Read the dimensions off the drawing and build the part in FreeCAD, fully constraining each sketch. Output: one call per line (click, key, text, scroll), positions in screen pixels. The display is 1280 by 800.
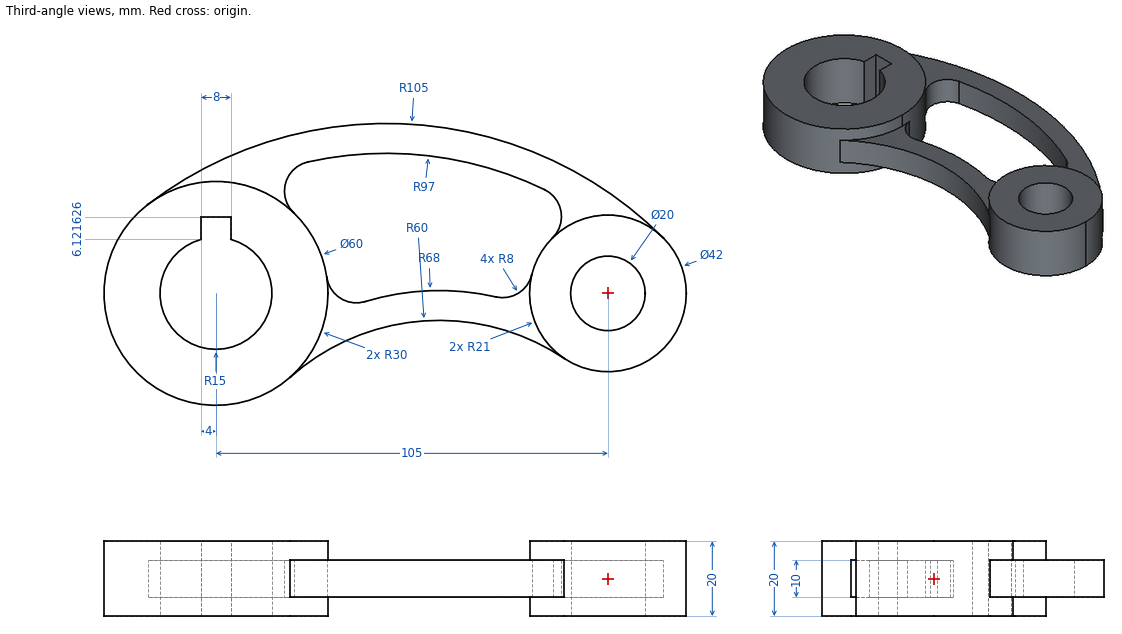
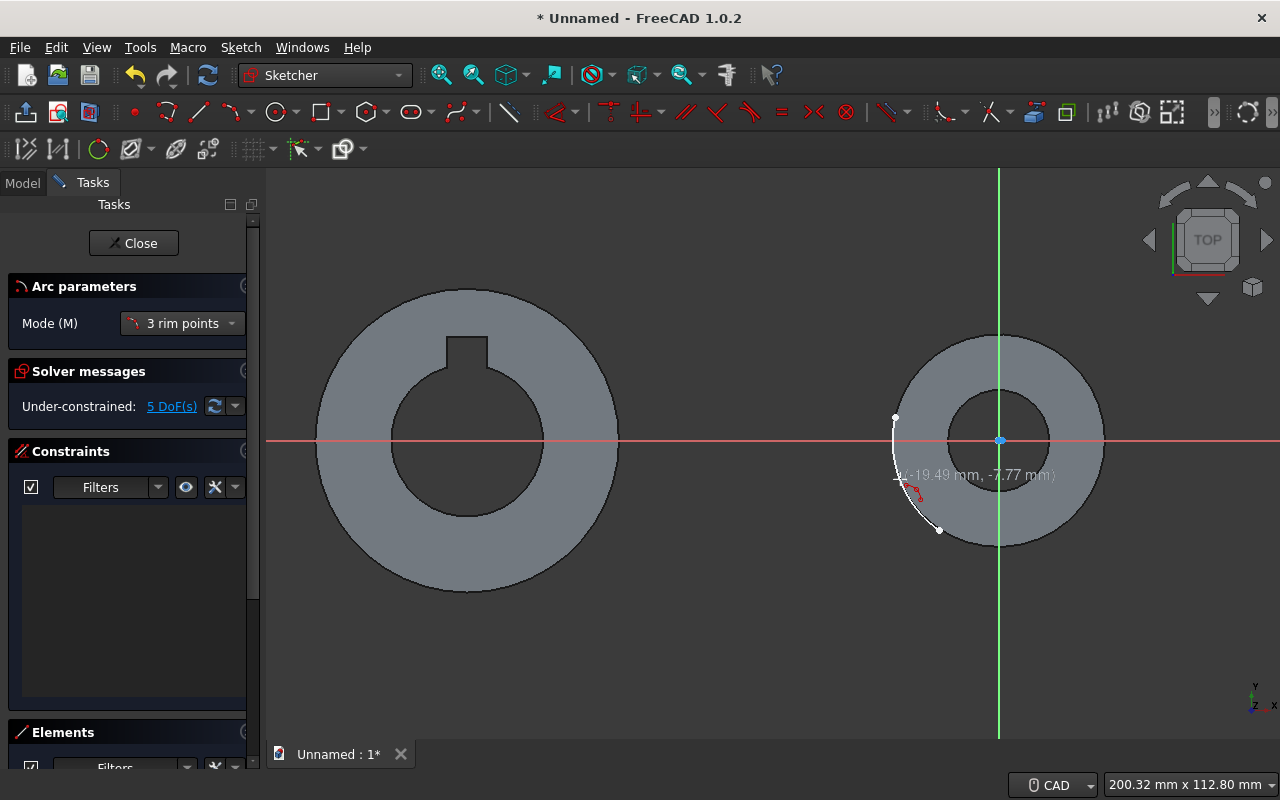
click(895, 418)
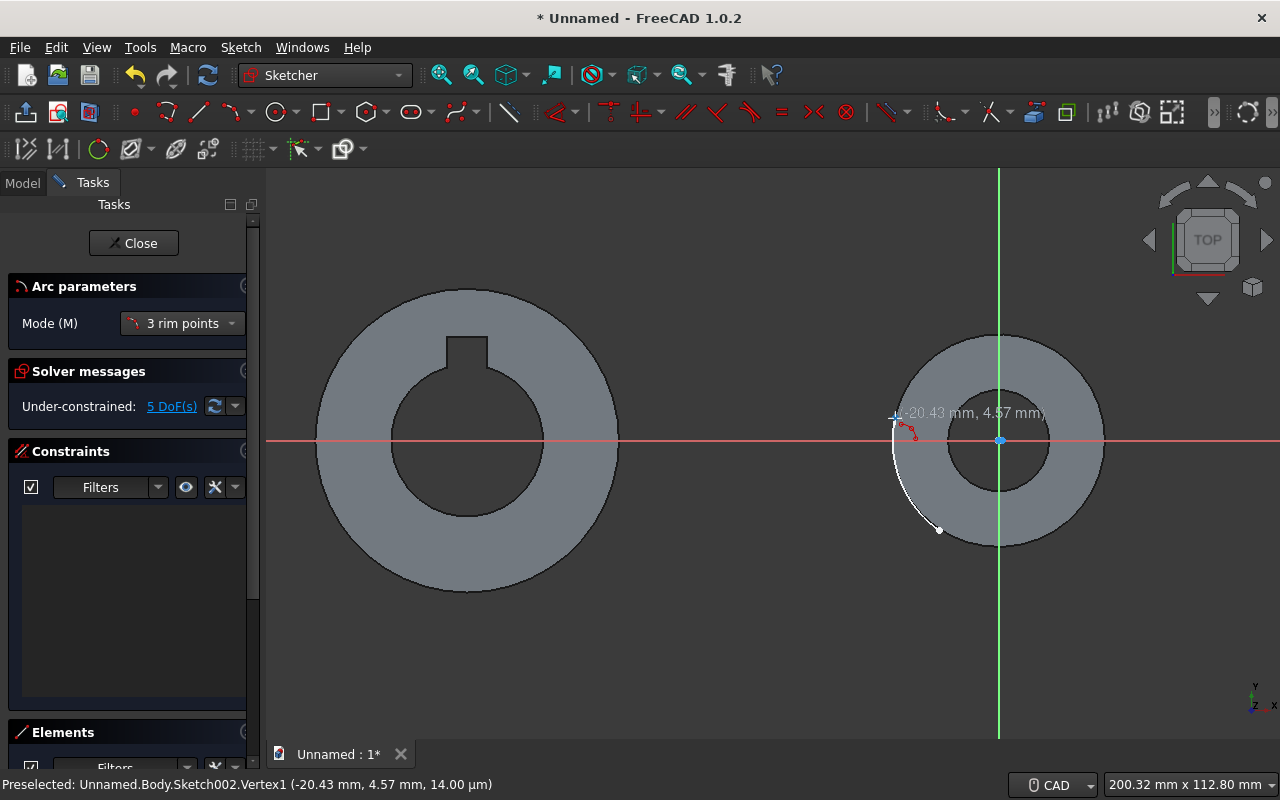
scroll(847, 446, up, 6)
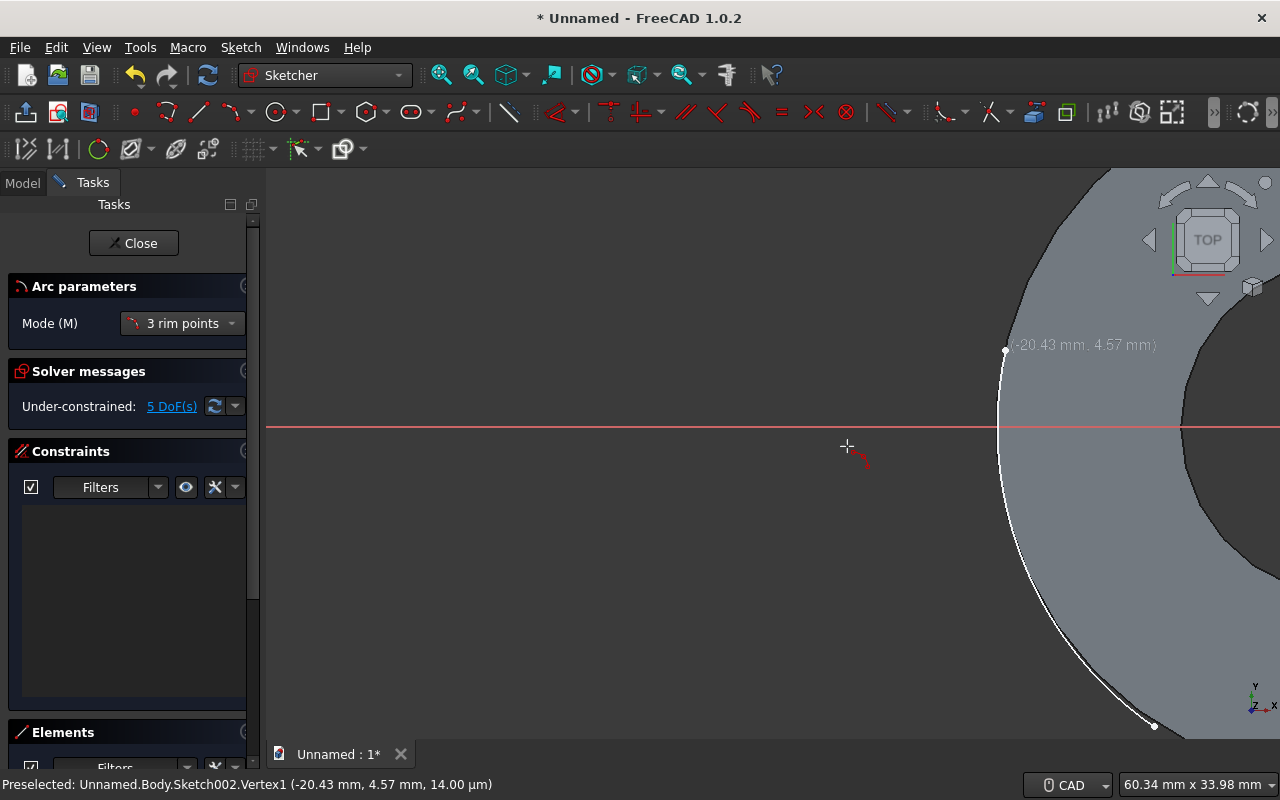
click(845, 443)
click(978, 399)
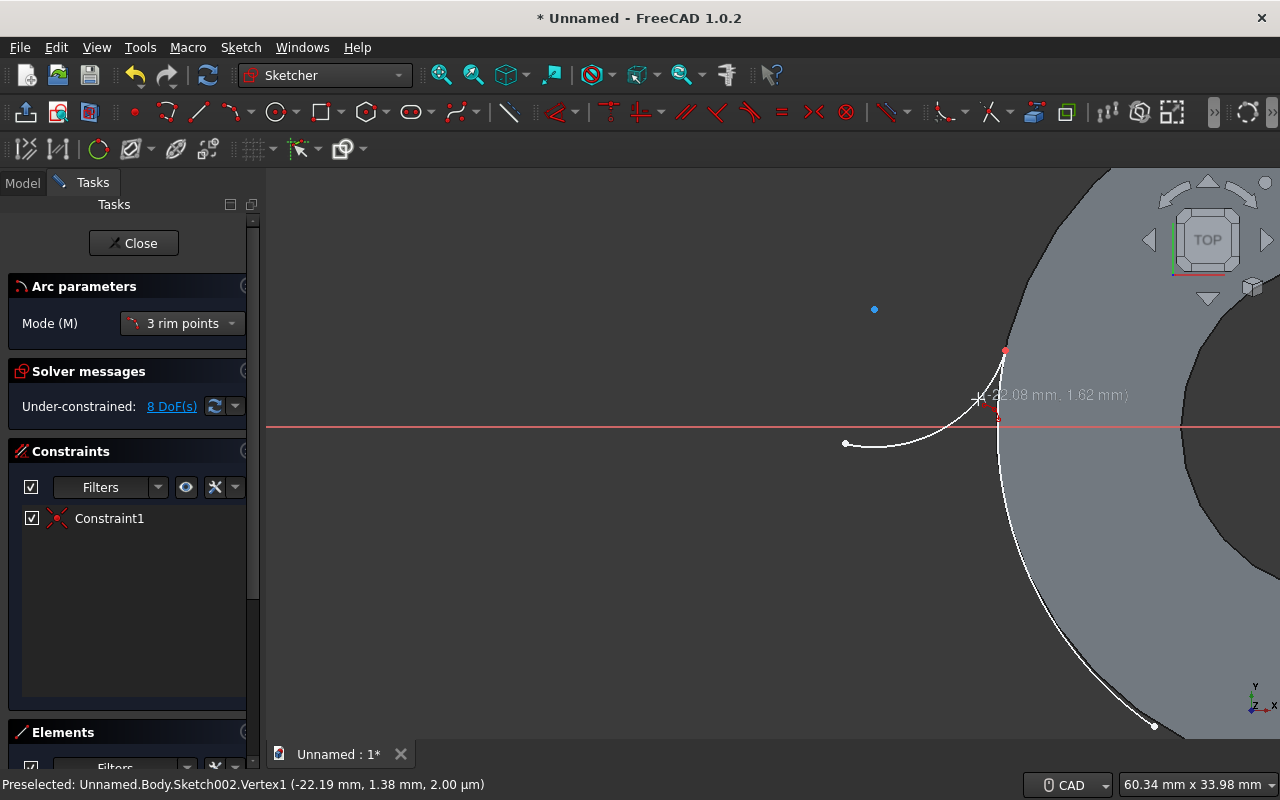
click(845, 444)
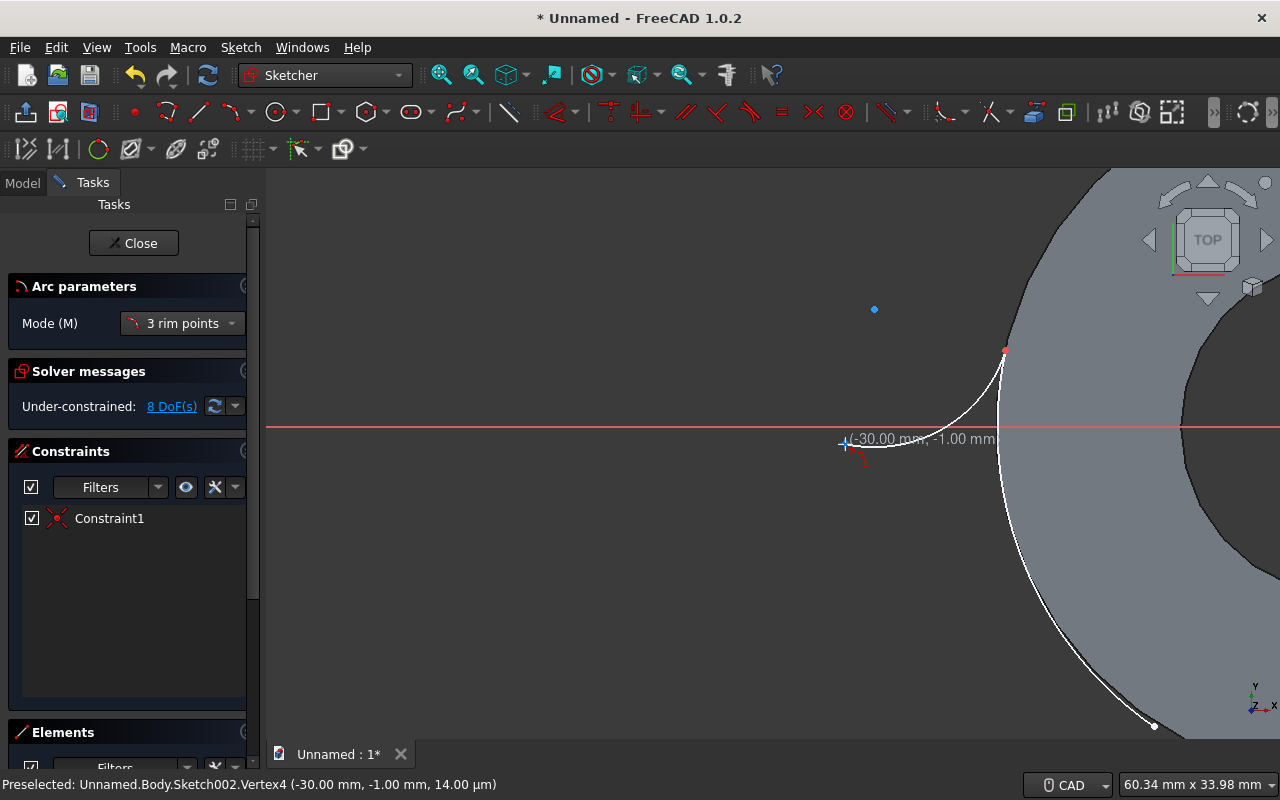
scroll(792, 525, down, 7)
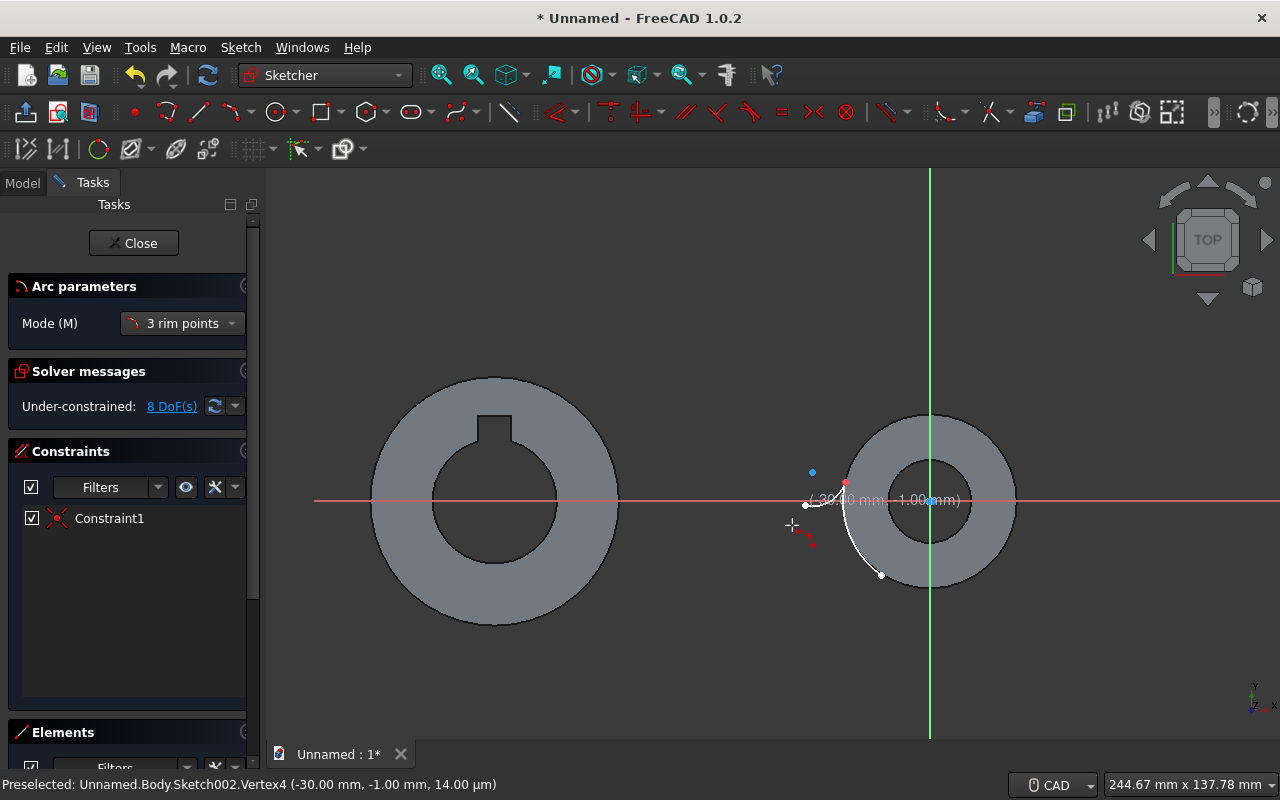
scroll(660, 511, up, 3)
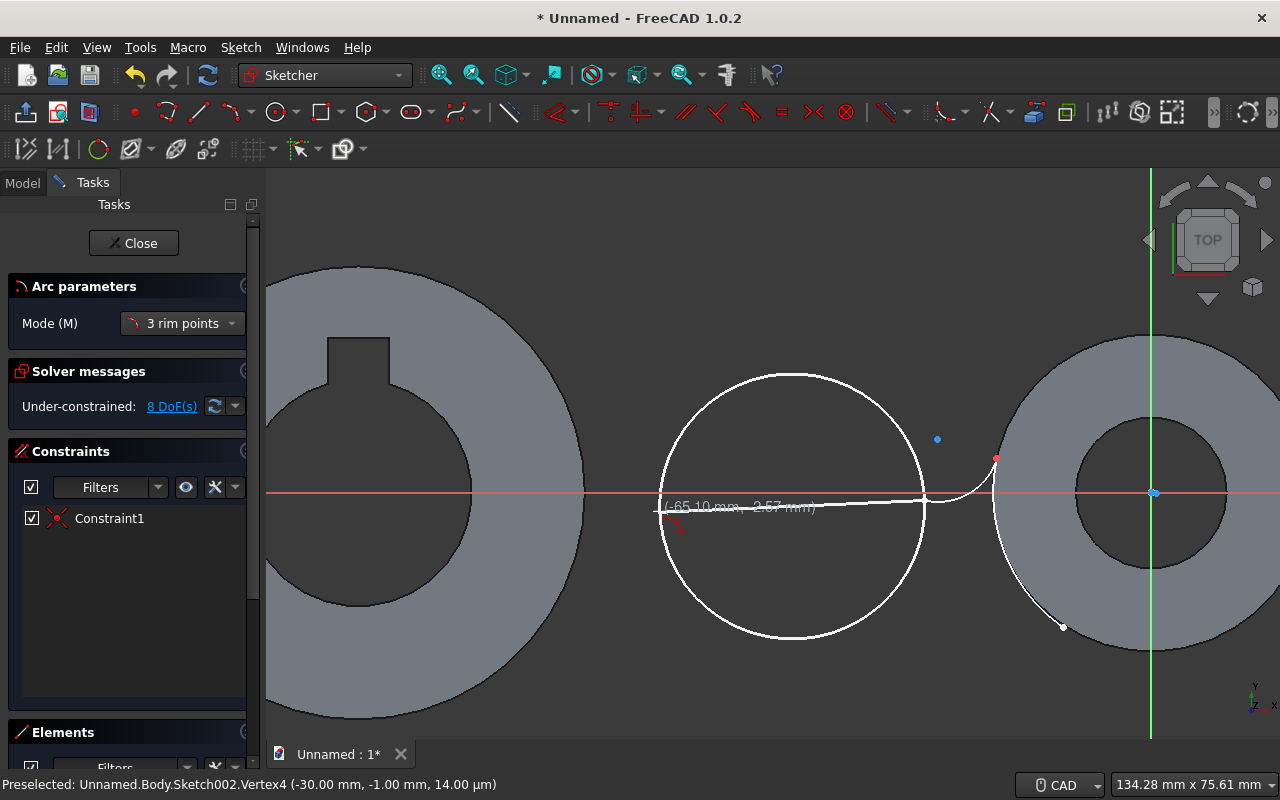
click(660, 510)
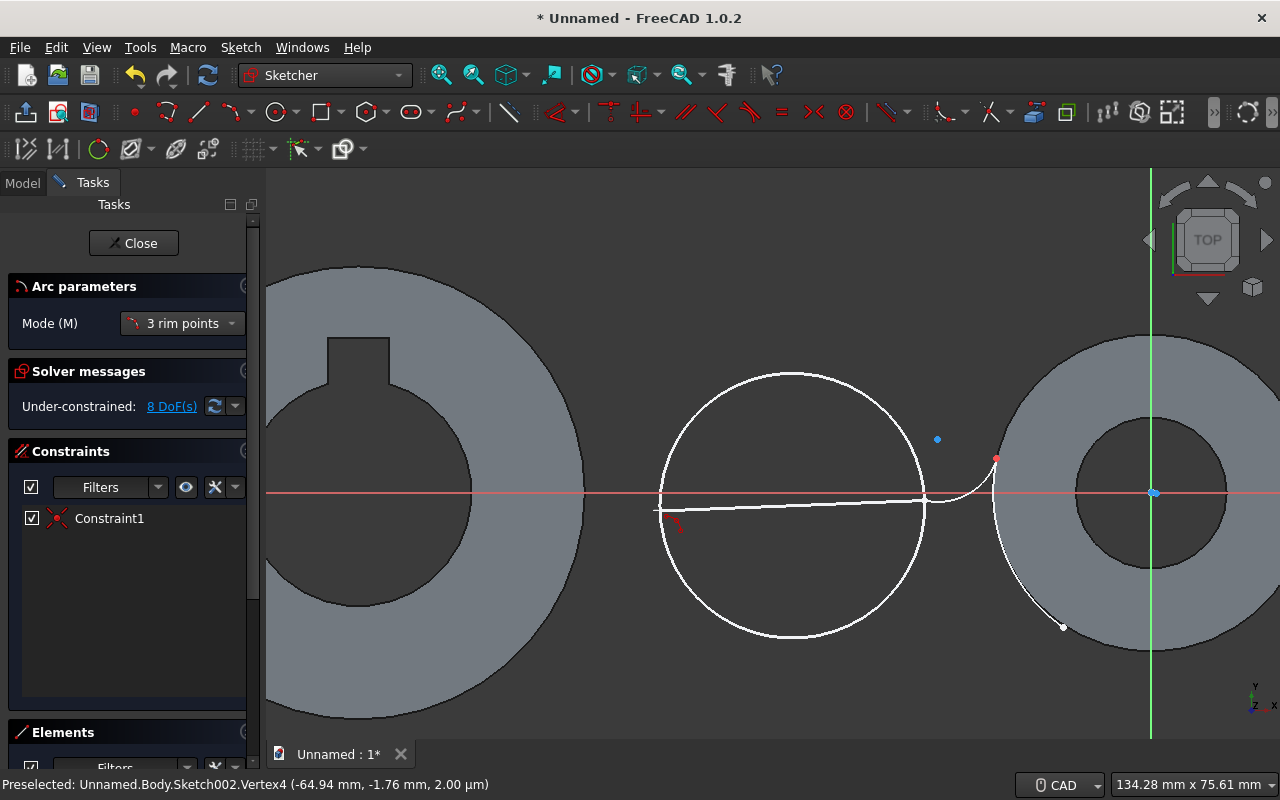
scroll(819, 487, up, 6)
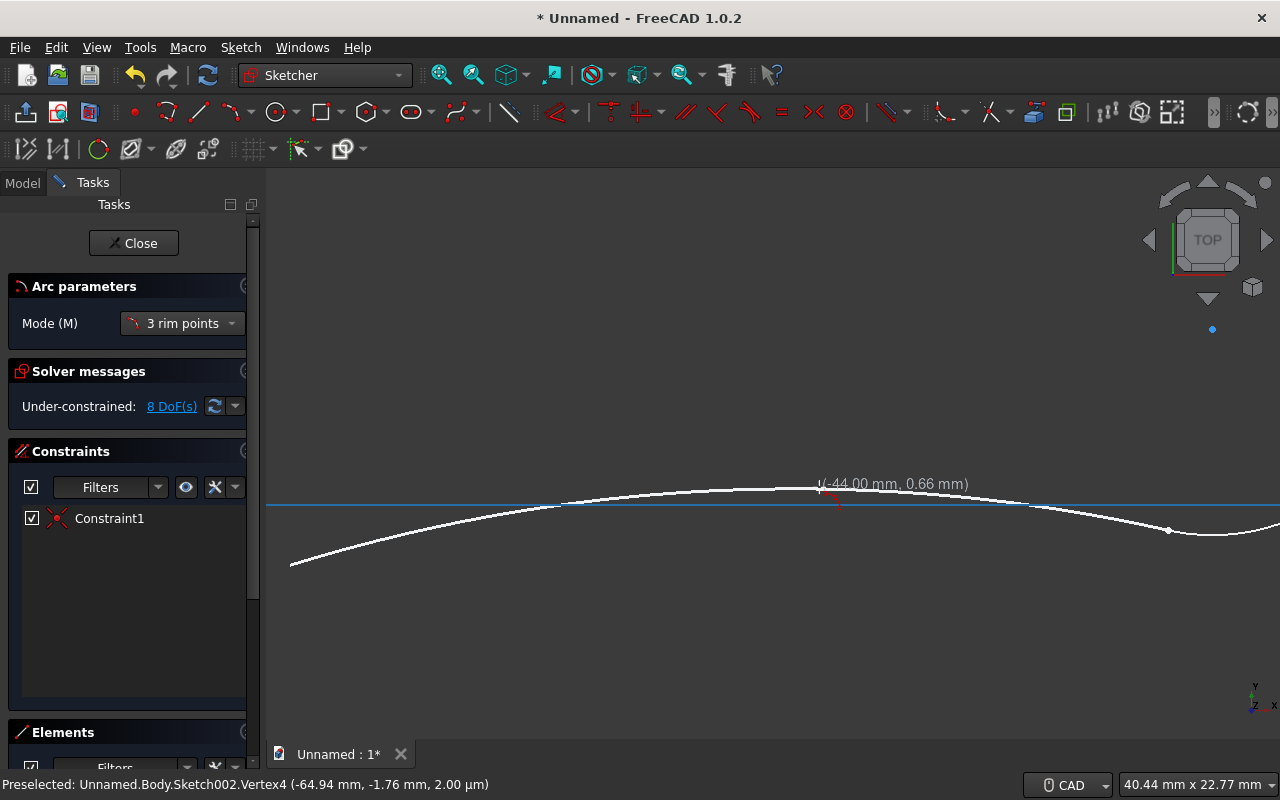
click(817, 487)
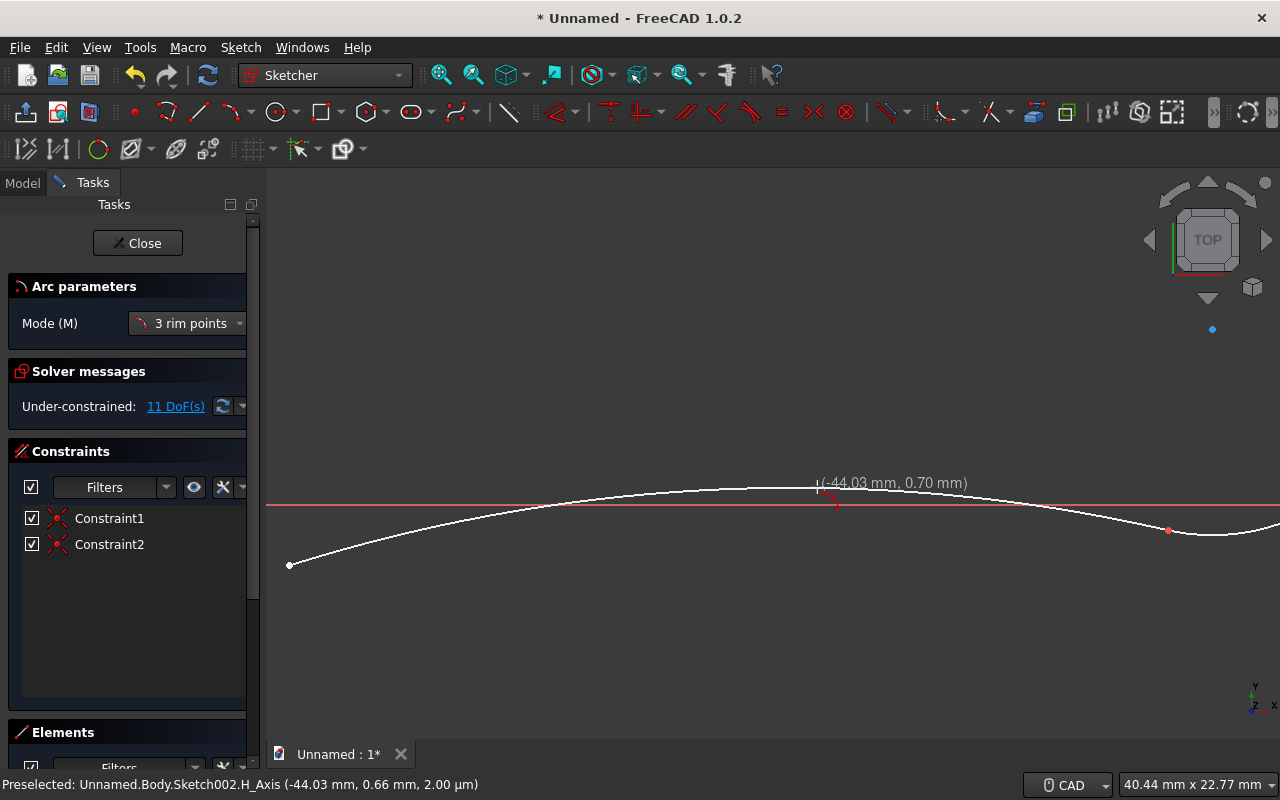
scroll(733, 500, down, 9)